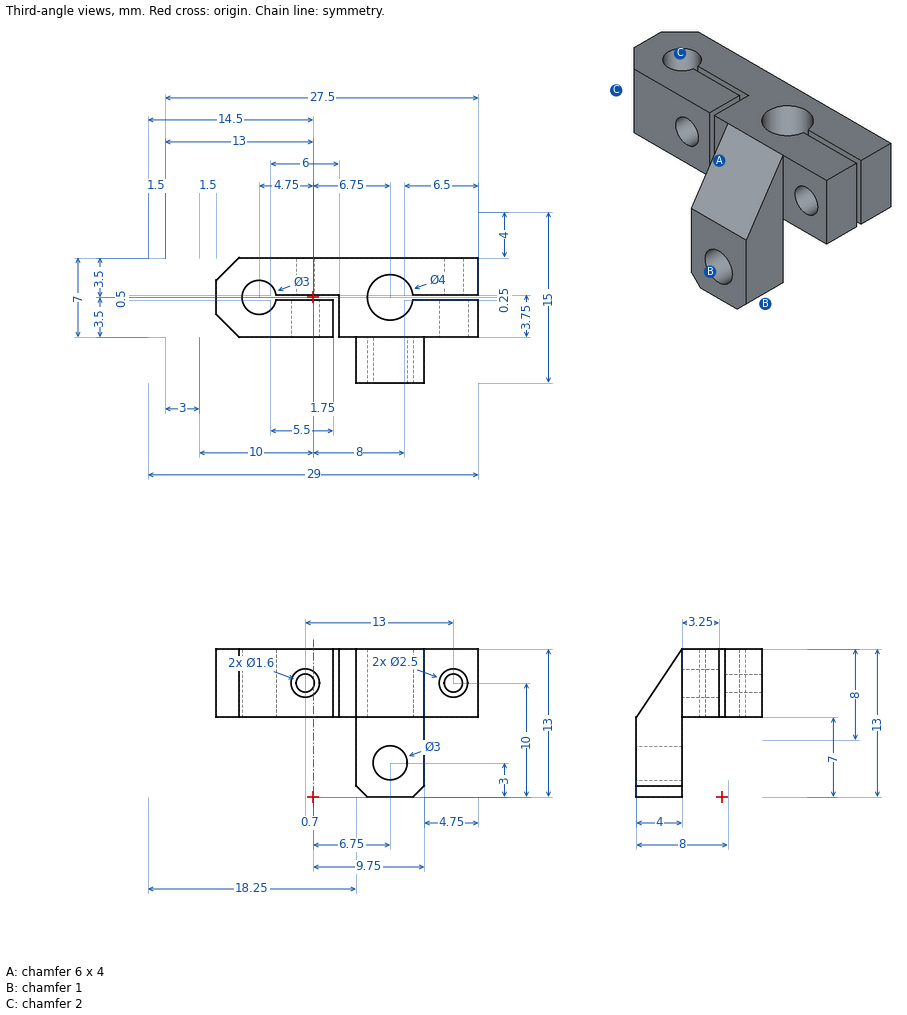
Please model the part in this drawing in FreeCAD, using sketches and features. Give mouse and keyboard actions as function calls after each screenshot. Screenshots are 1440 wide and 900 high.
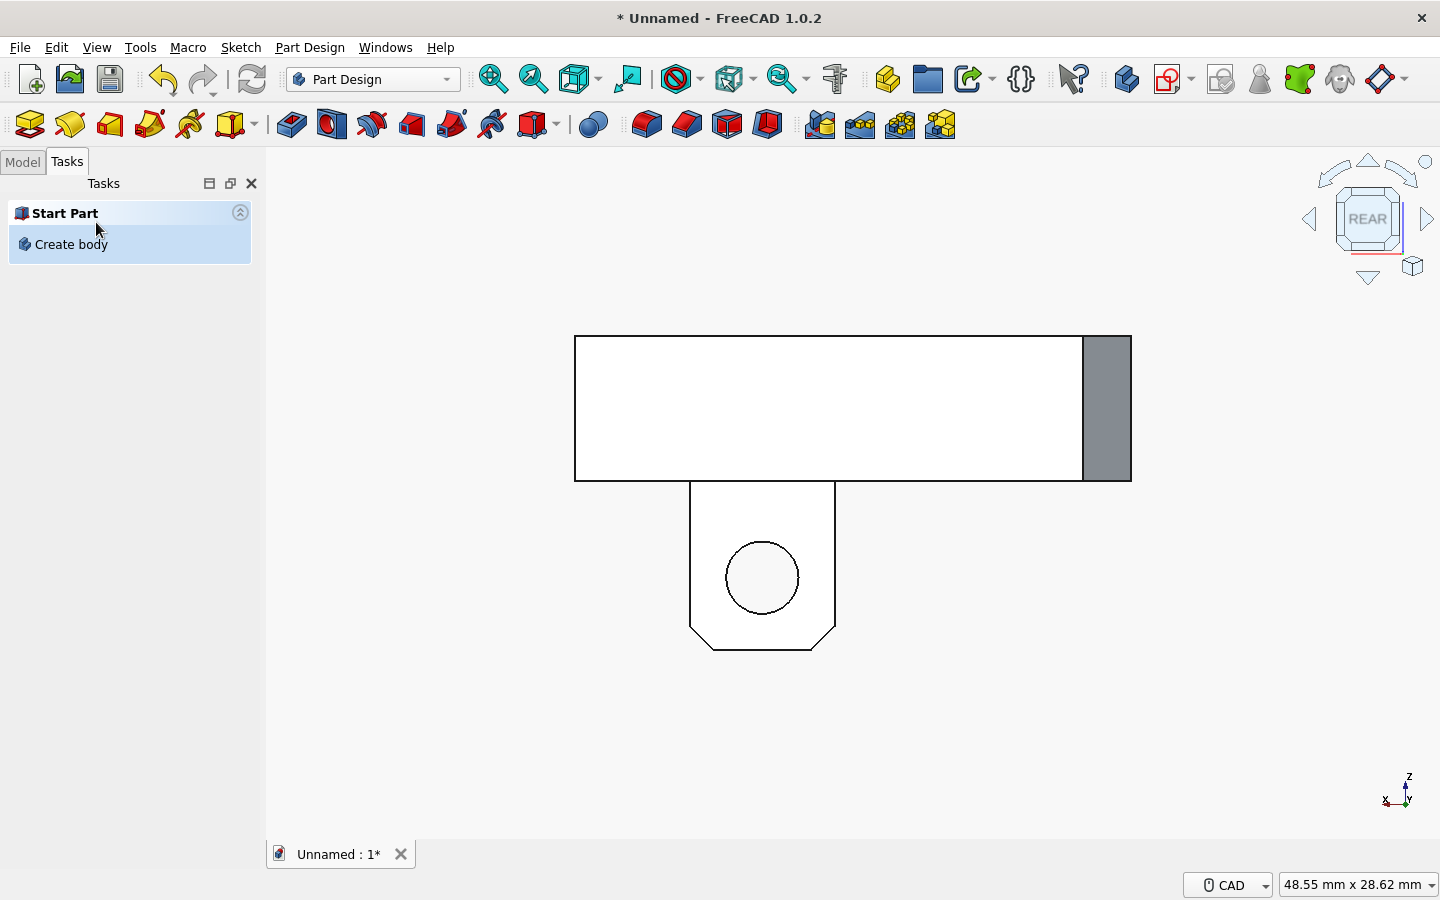
click(684, 407)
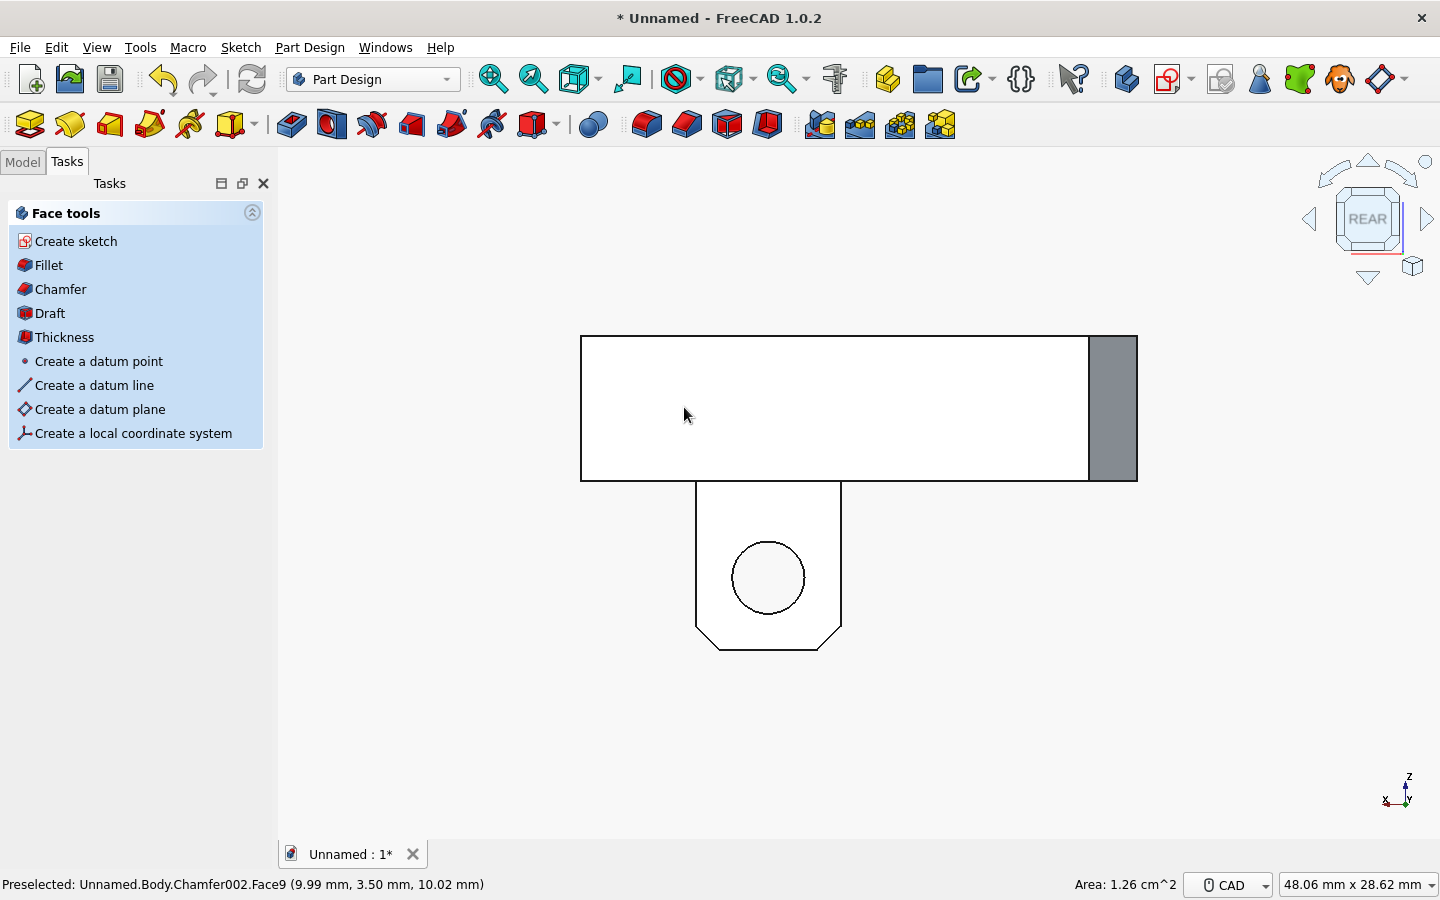
click(1168, 80)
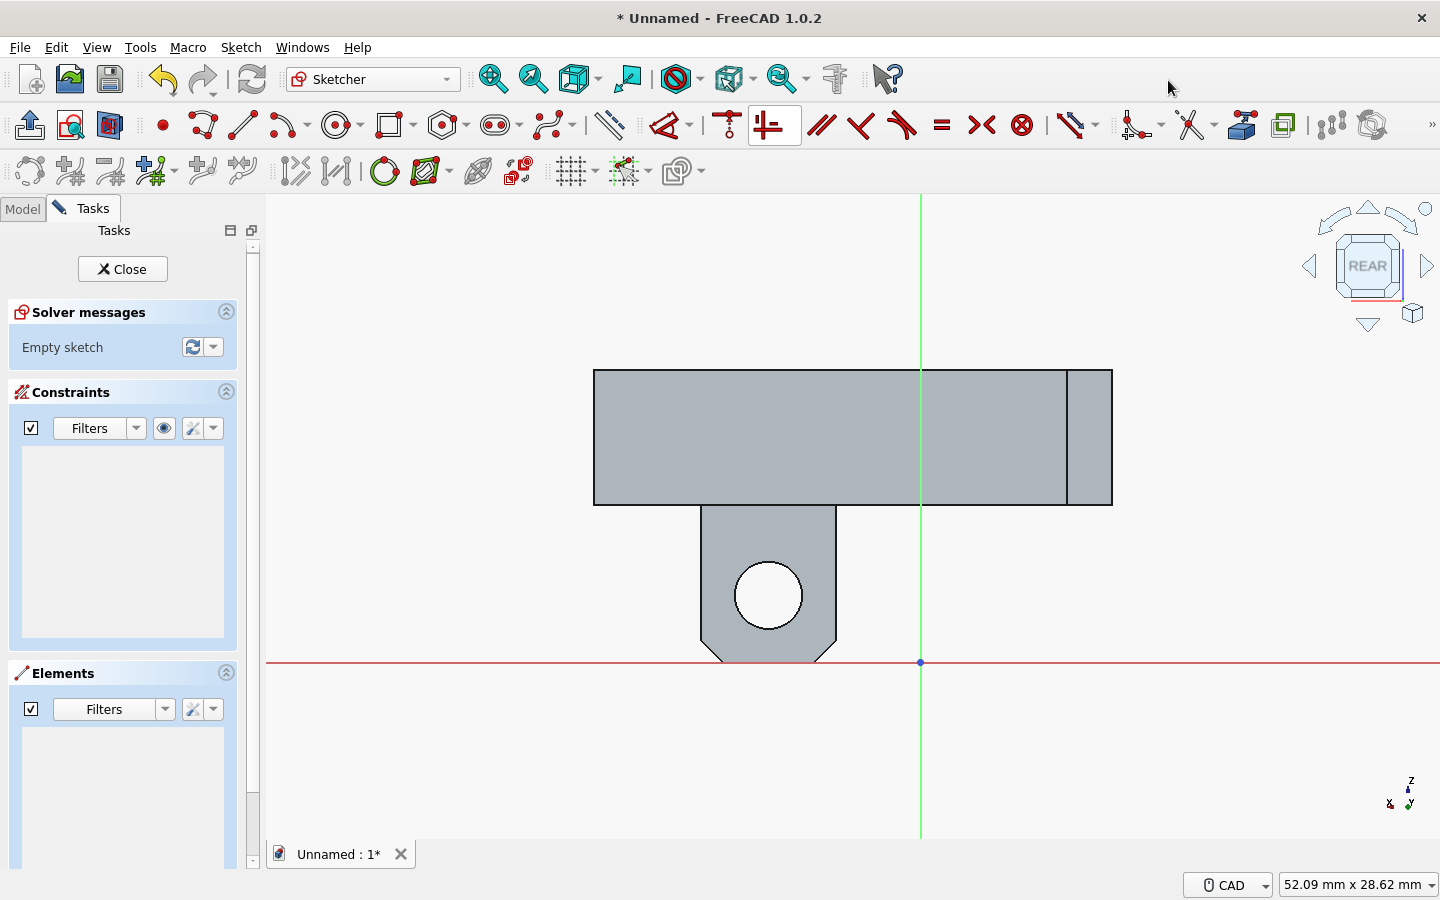
scroll(796, 571, up, 3)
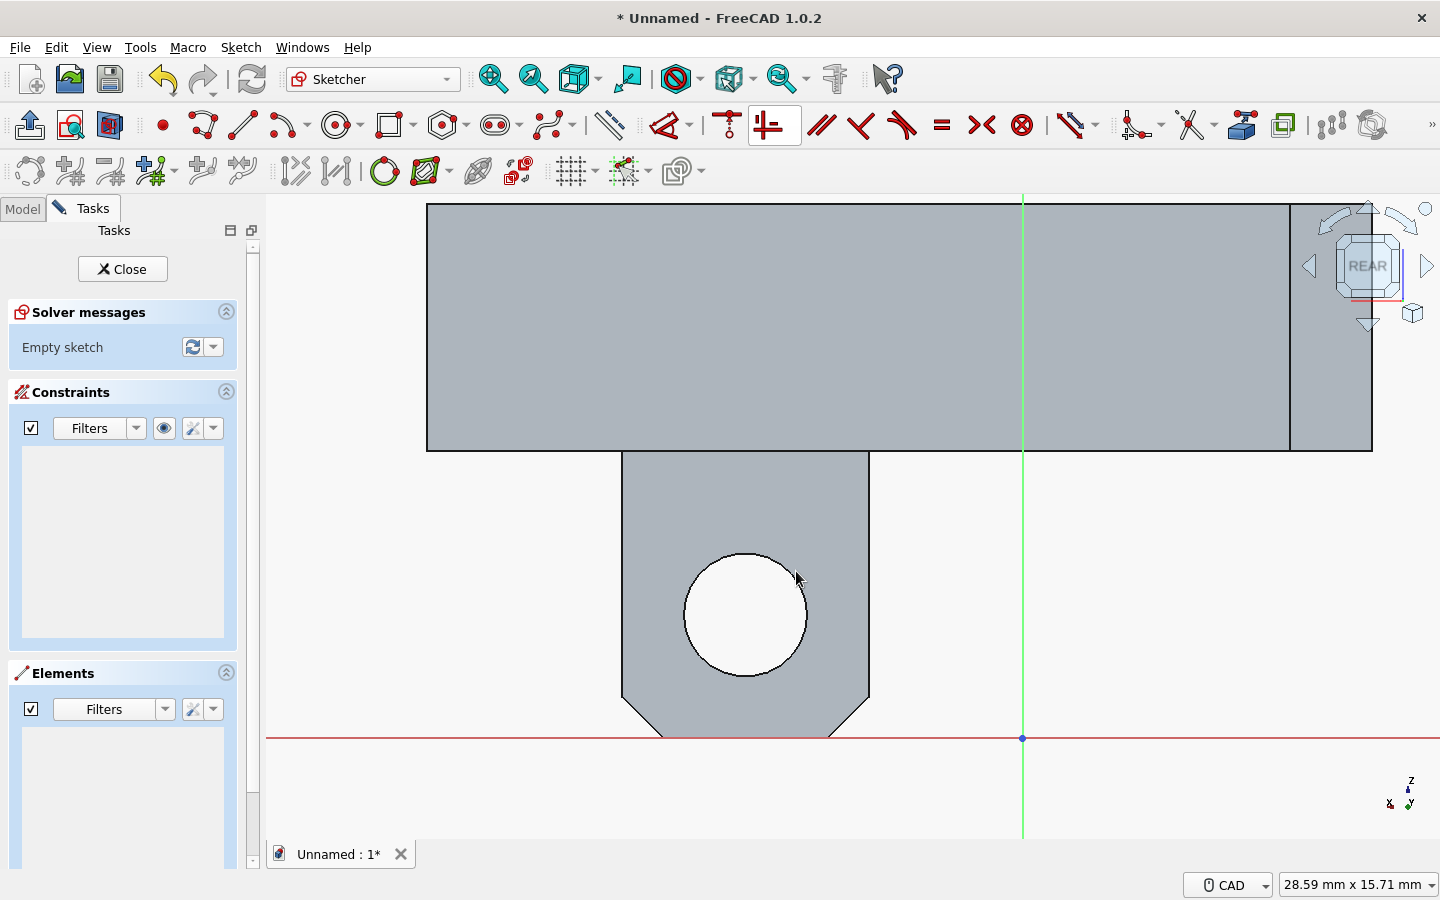
click(336, 126)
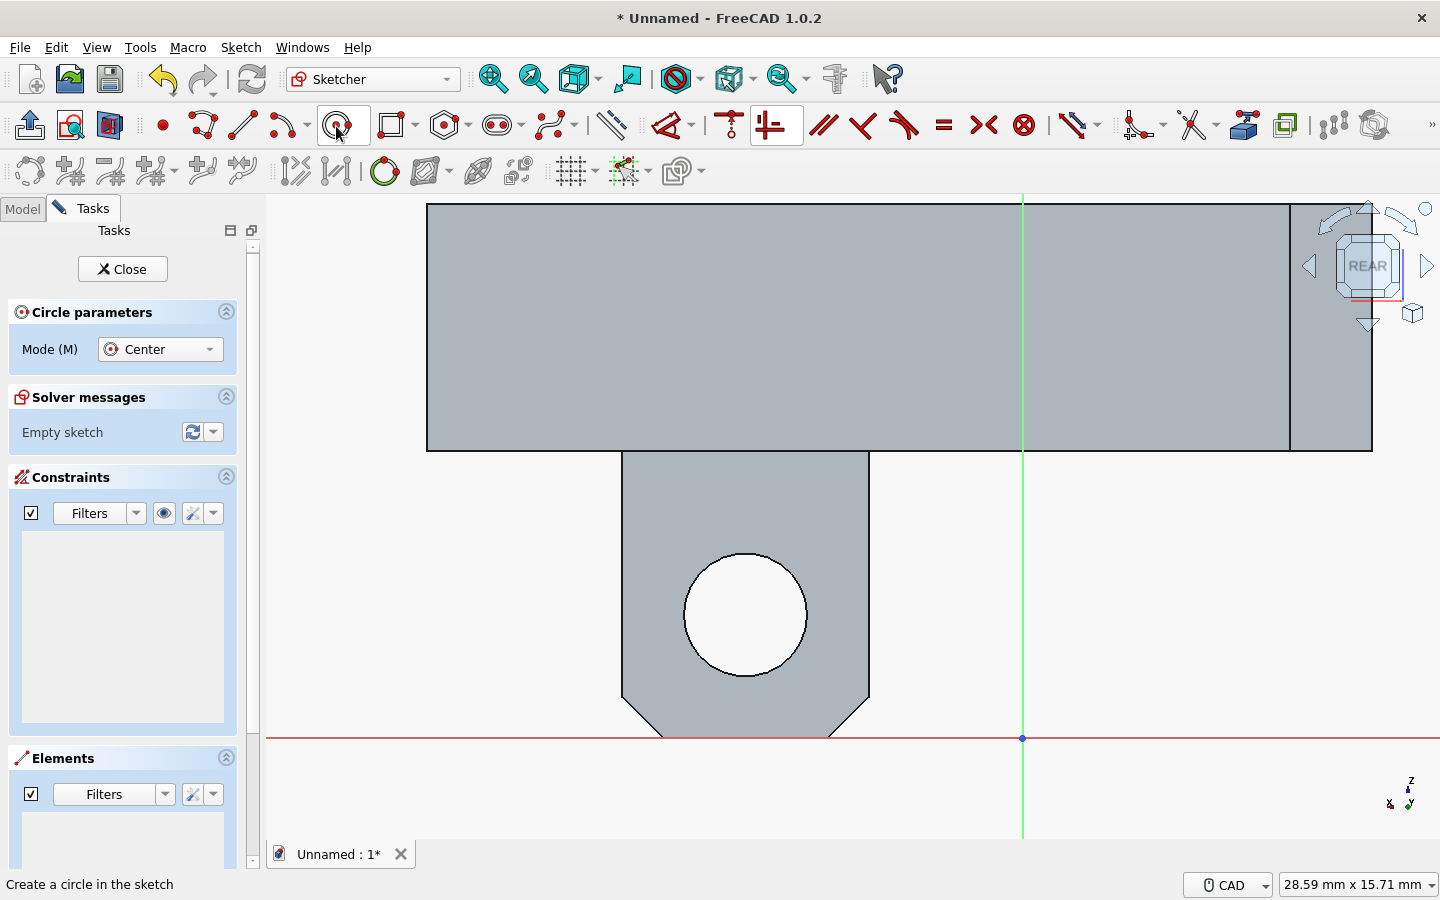
click(1051, 327)
move(1075, 304)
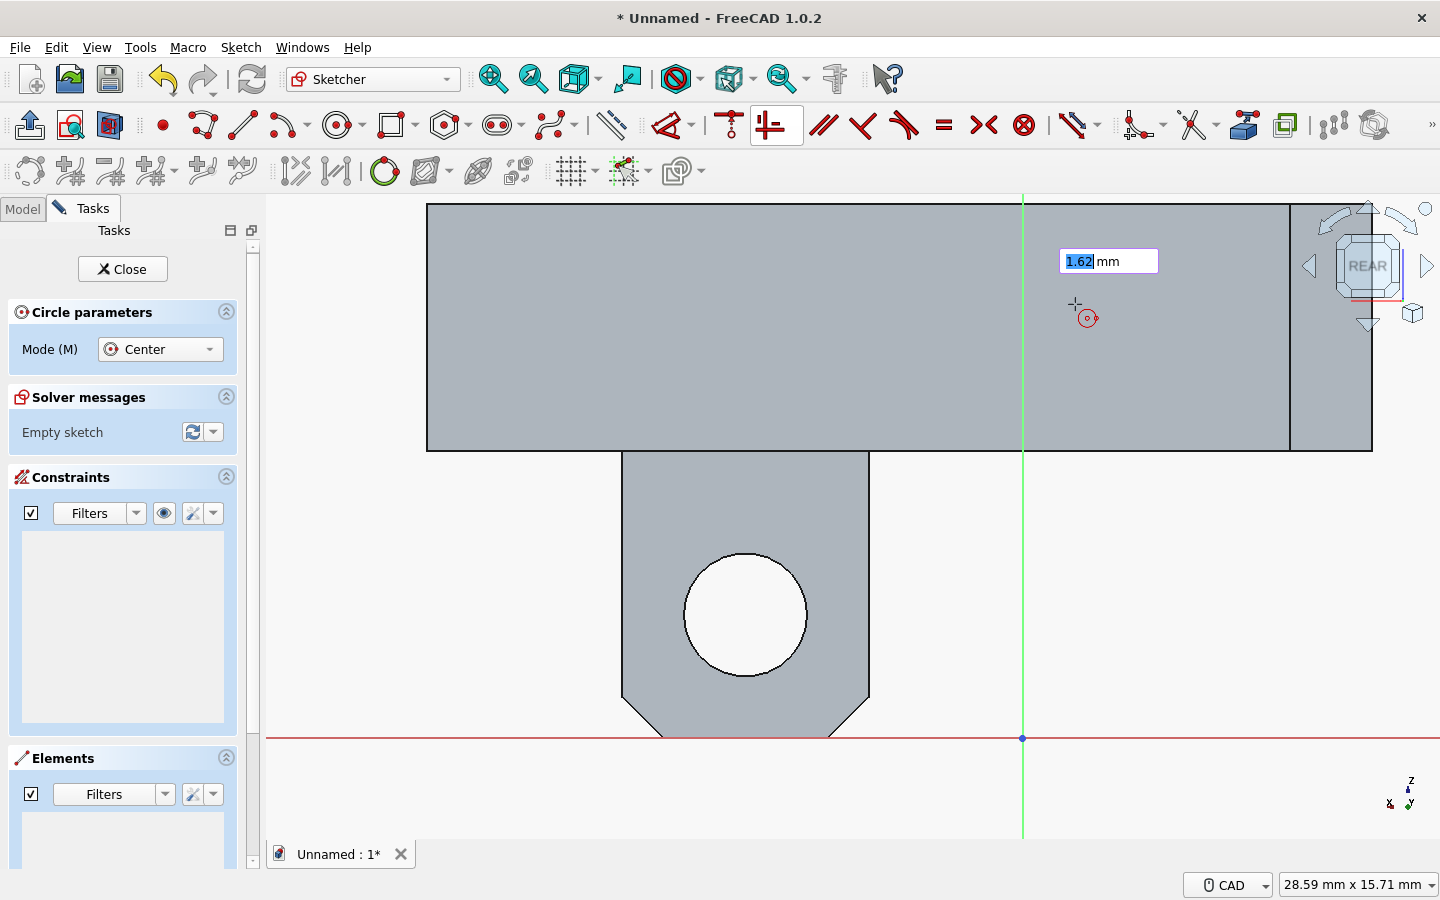
text(1.6)
key(Return)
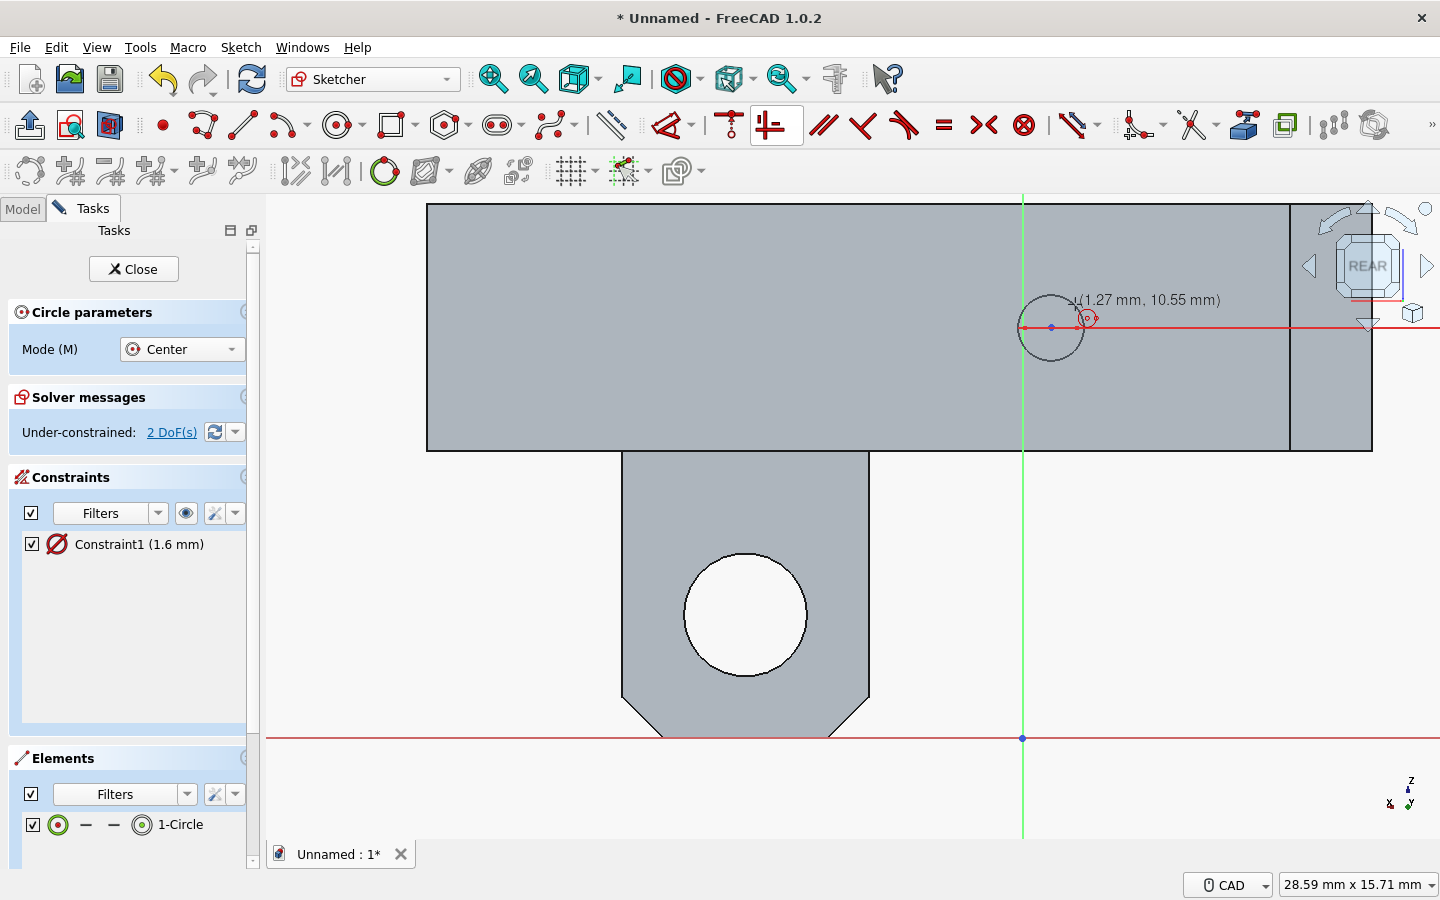
click(518, 327)
move(541, 304)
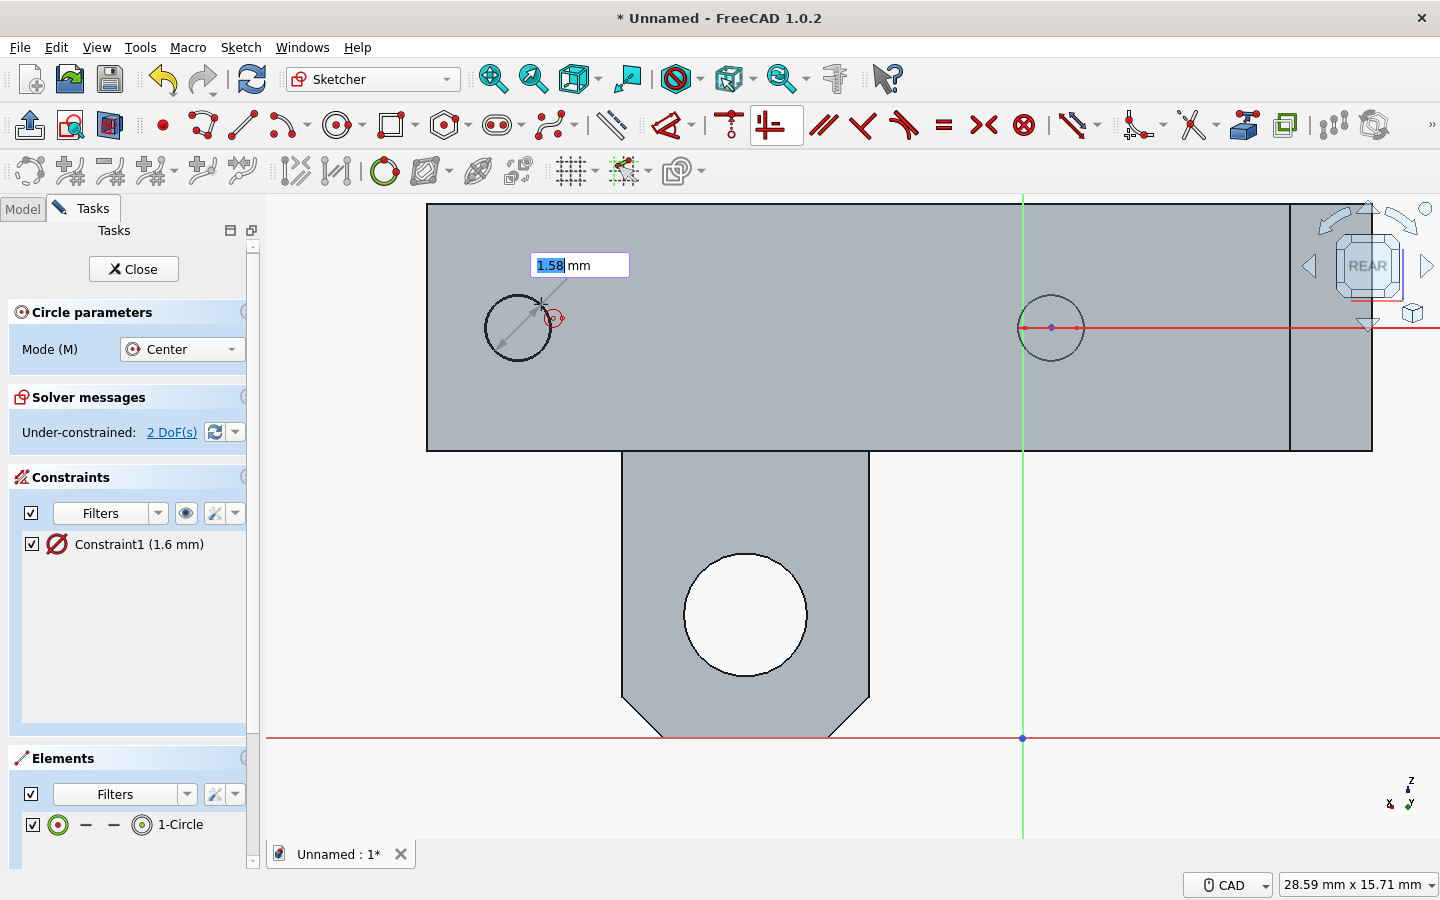
text(1.6)
key(Return)
key(Escape)